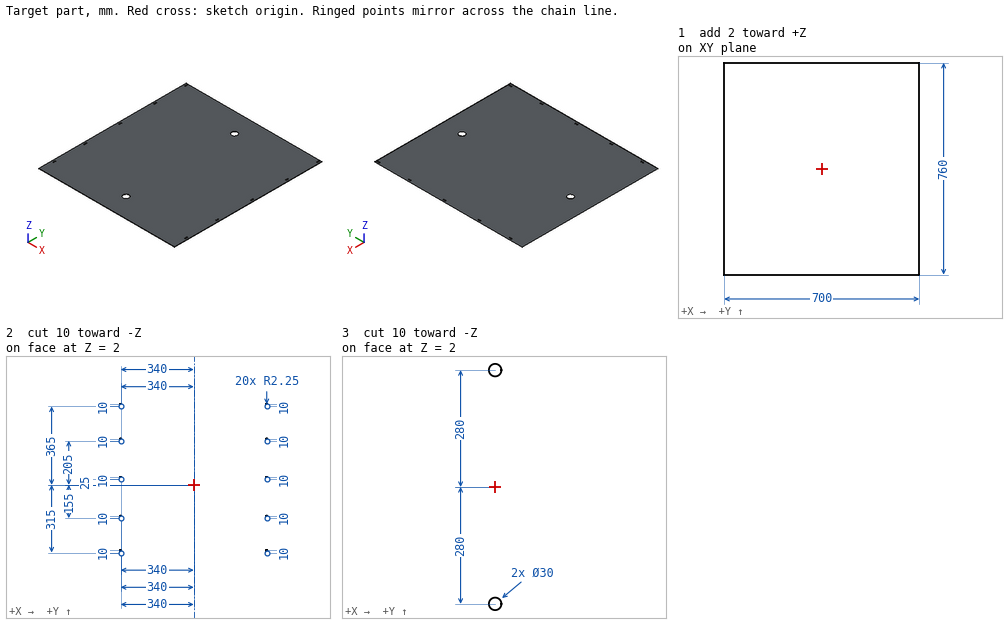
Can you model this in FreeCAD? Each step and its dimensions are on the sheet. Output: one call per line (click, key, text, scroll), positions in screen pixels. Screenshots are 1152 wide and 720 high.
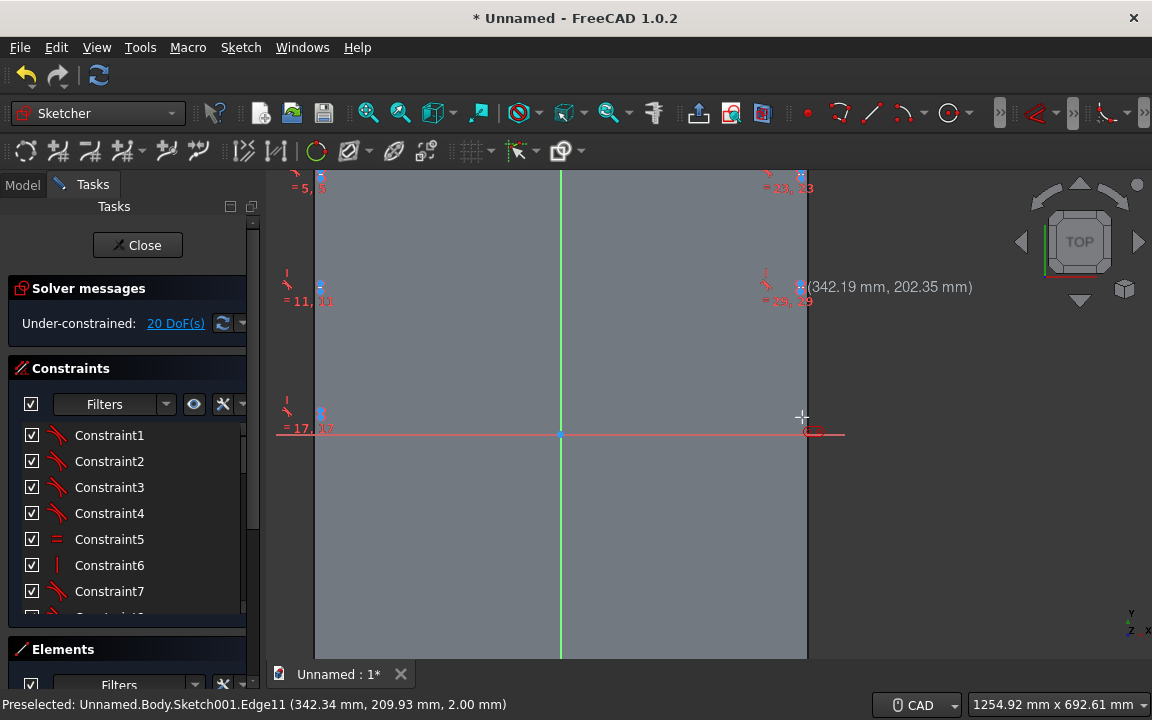
click(801, 417)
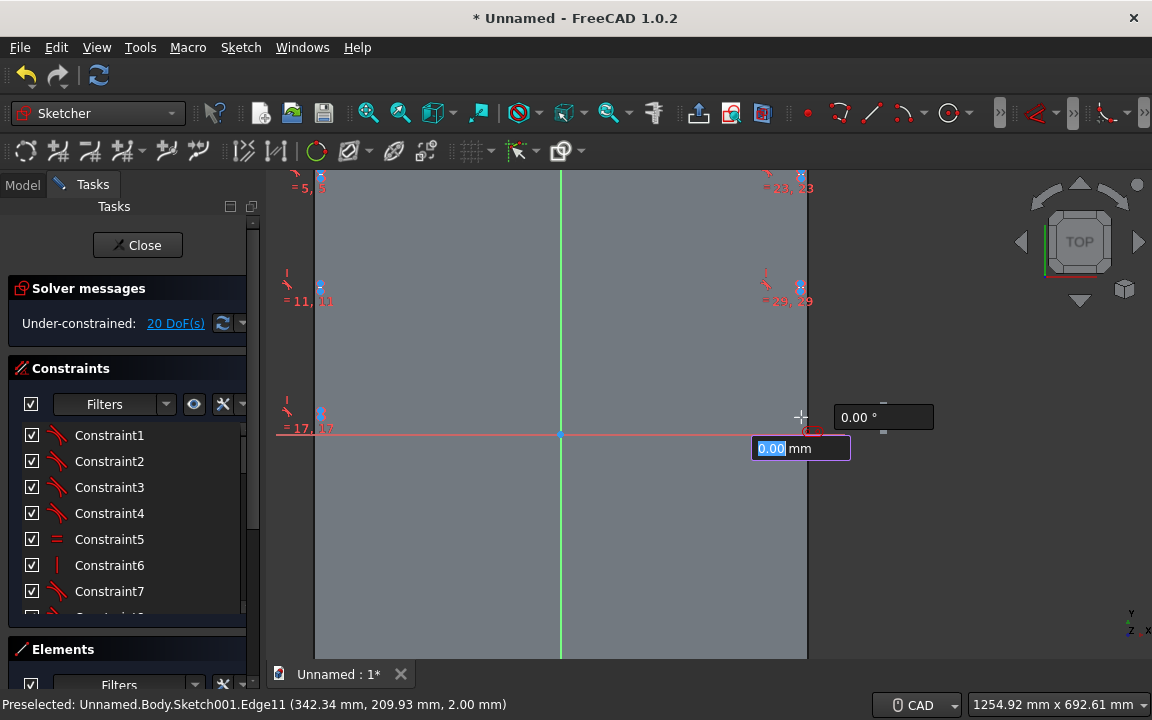
scroll(801, 410, up, 5)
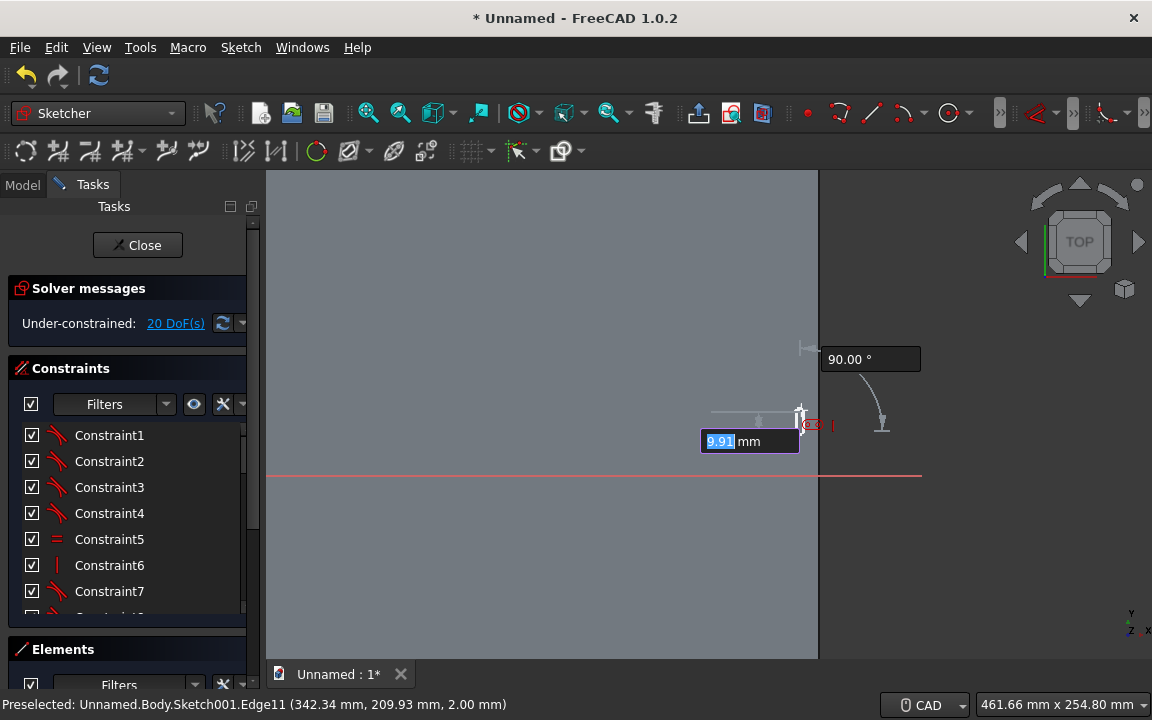
click(800, 409)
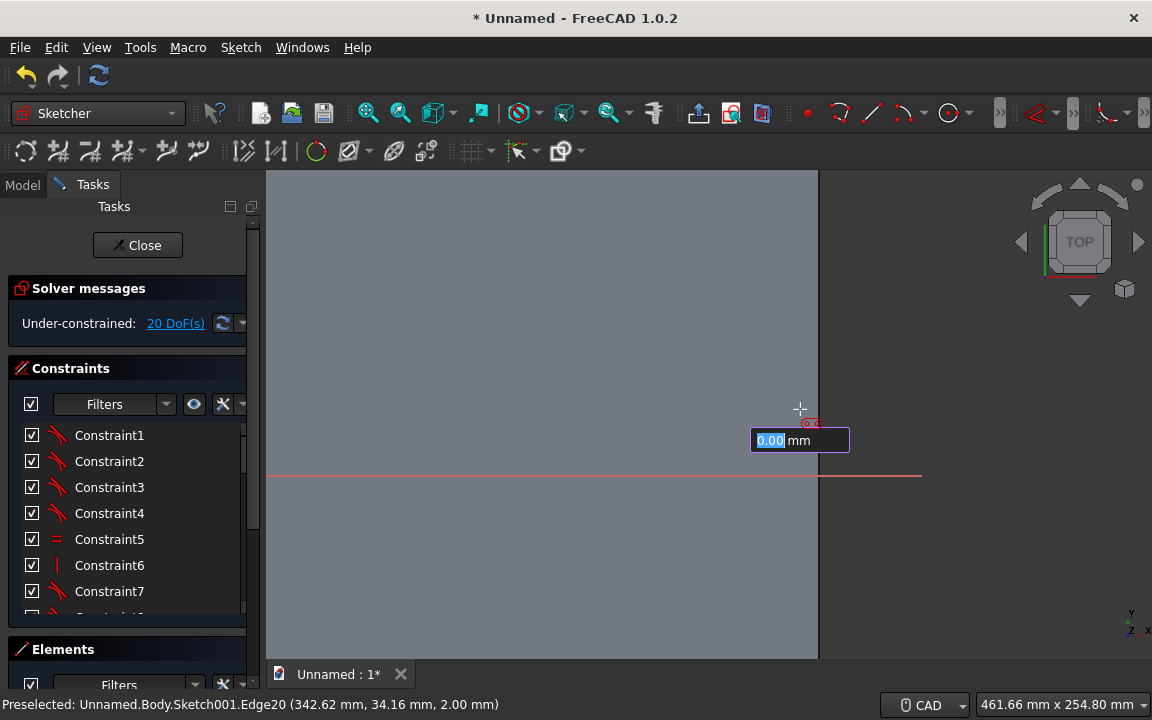
scroll(804, 418, up, 7)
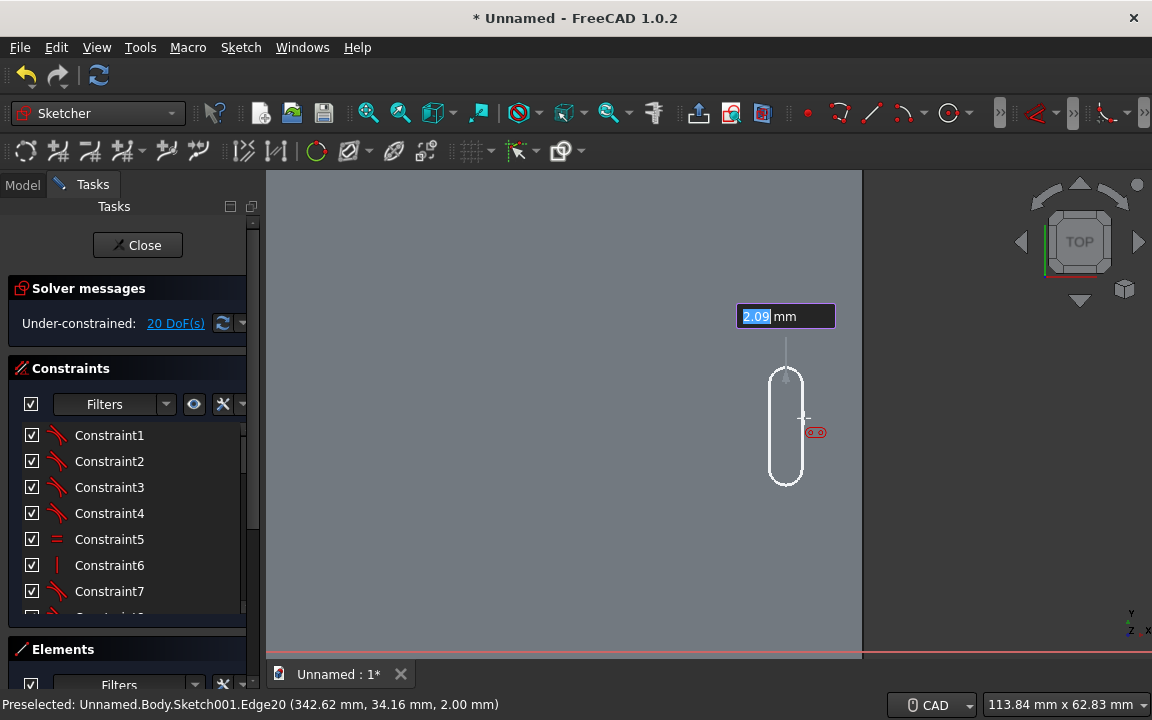
click(803, 418)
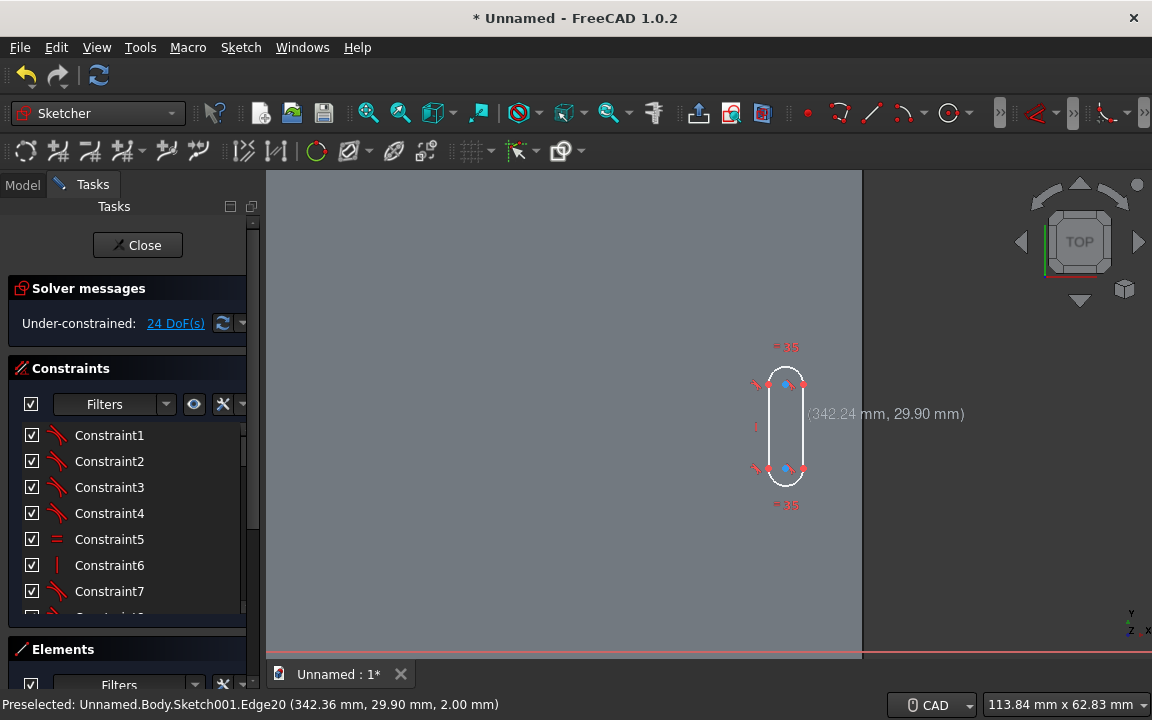
scroll(802, 414, down, 14)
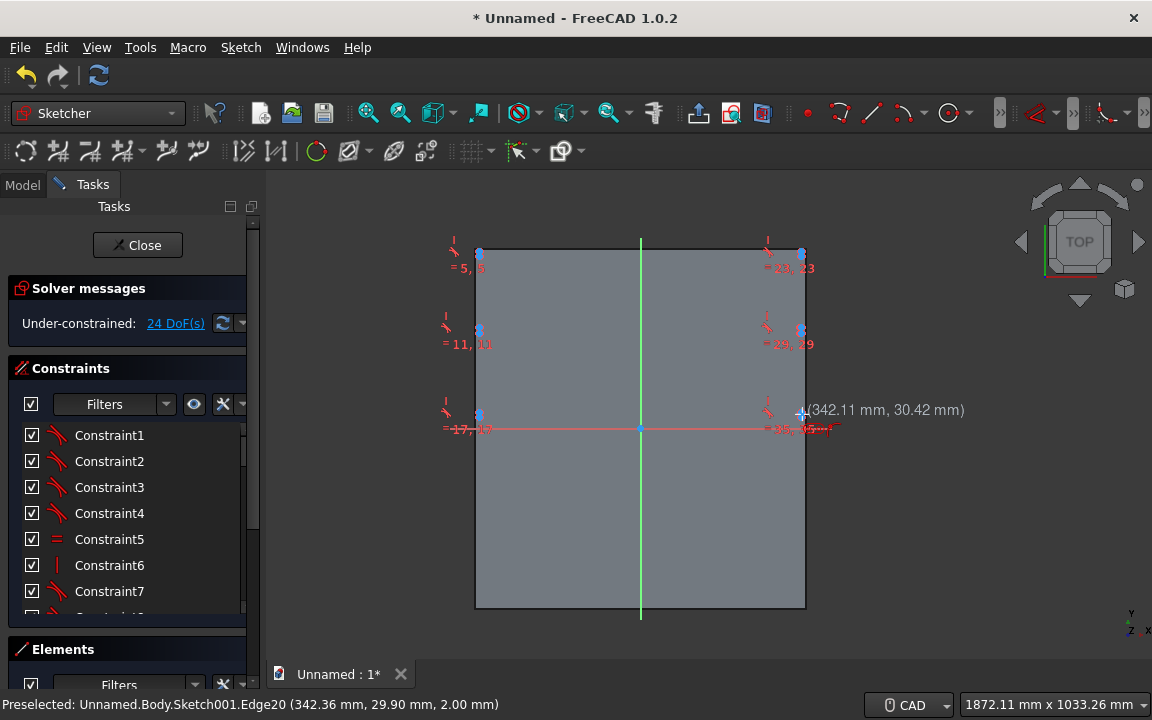
scroll(480, 578, up, 16)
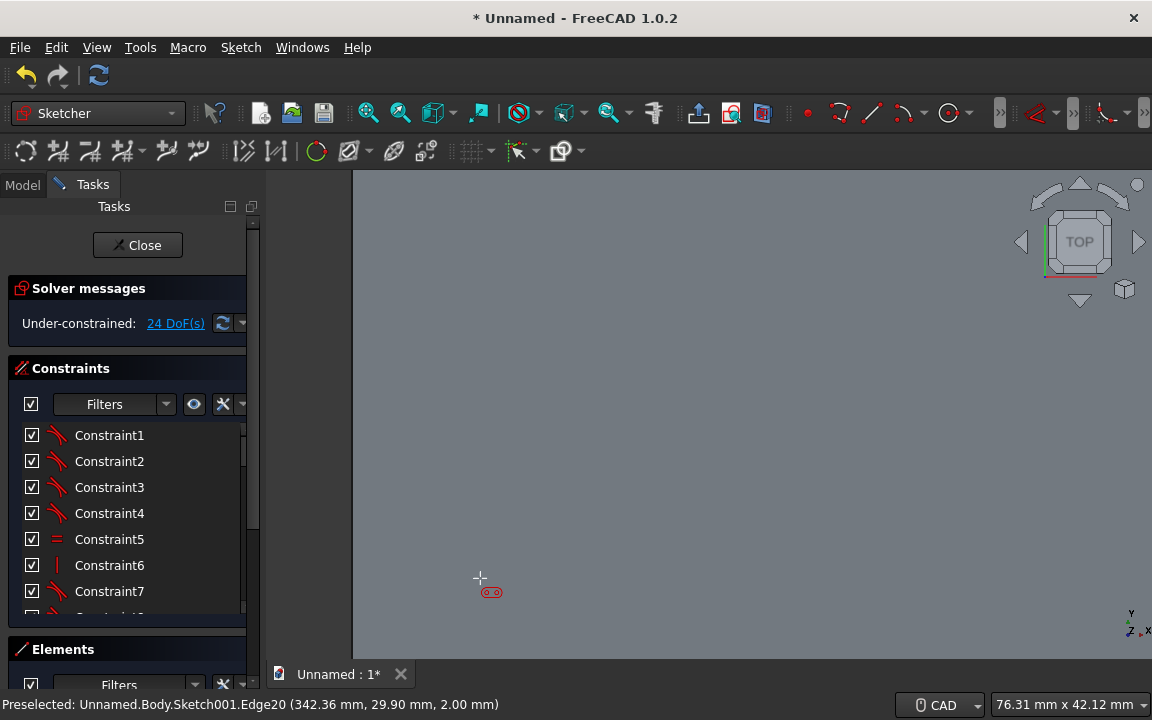
scroll(480, 579, down, 16)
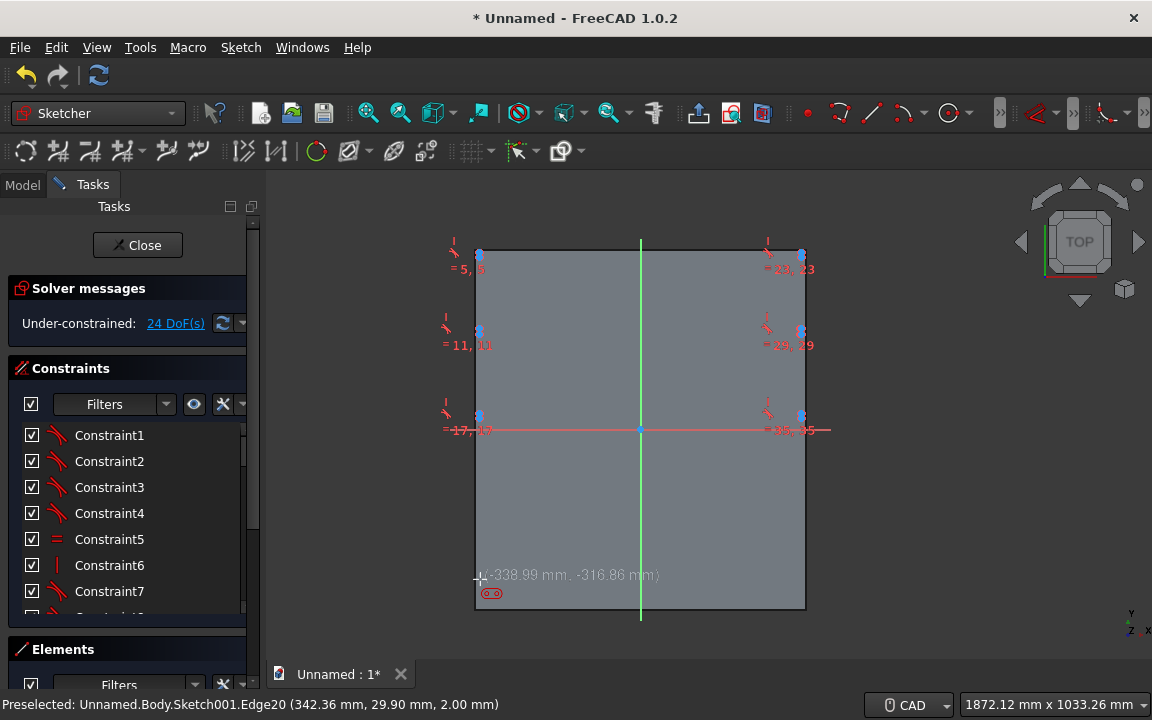
click(480, 579)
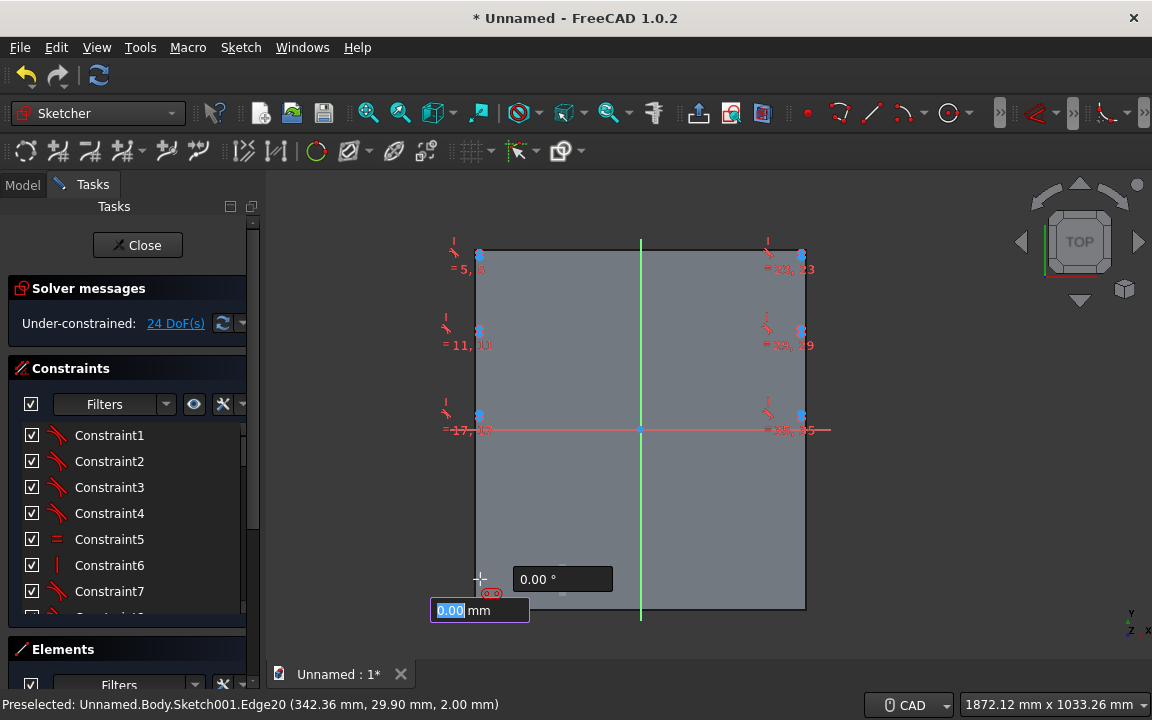
scroll(480, 574, up, 7)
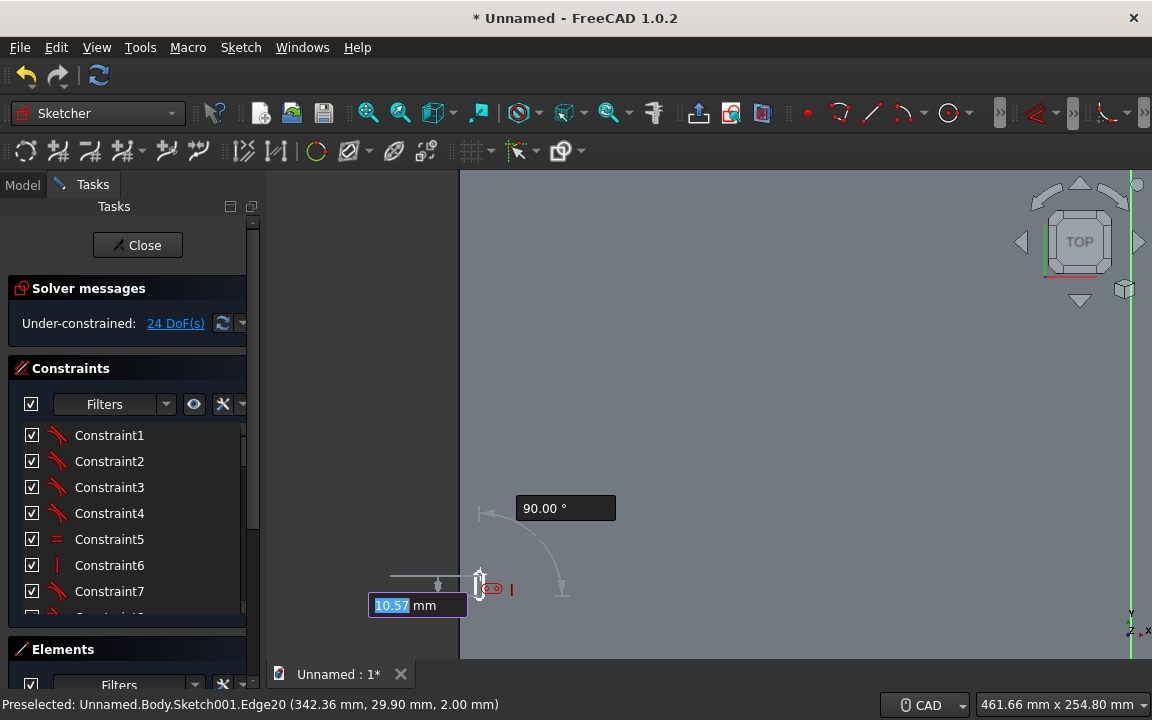
click(479, 572)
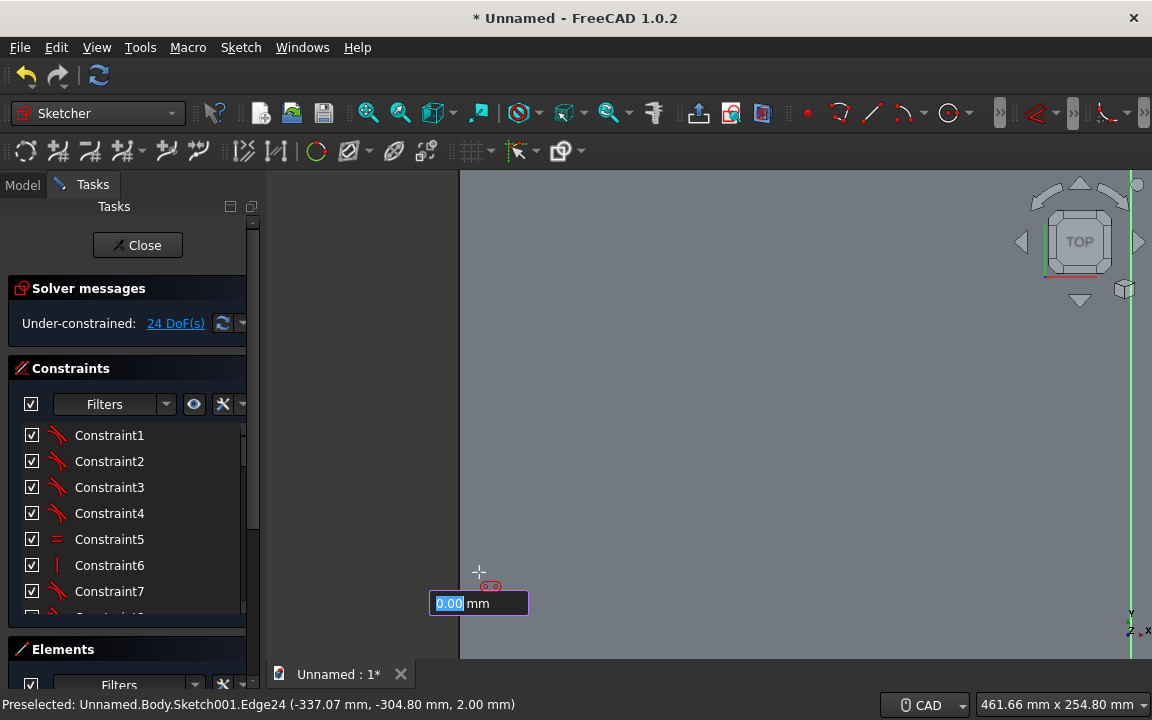
scroll(483, 582, up, 7)